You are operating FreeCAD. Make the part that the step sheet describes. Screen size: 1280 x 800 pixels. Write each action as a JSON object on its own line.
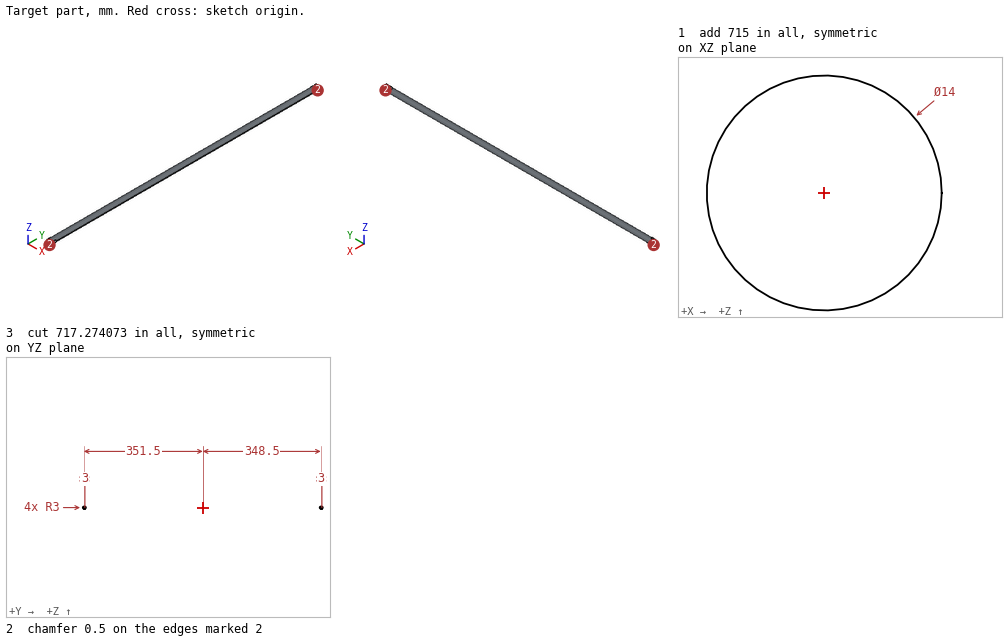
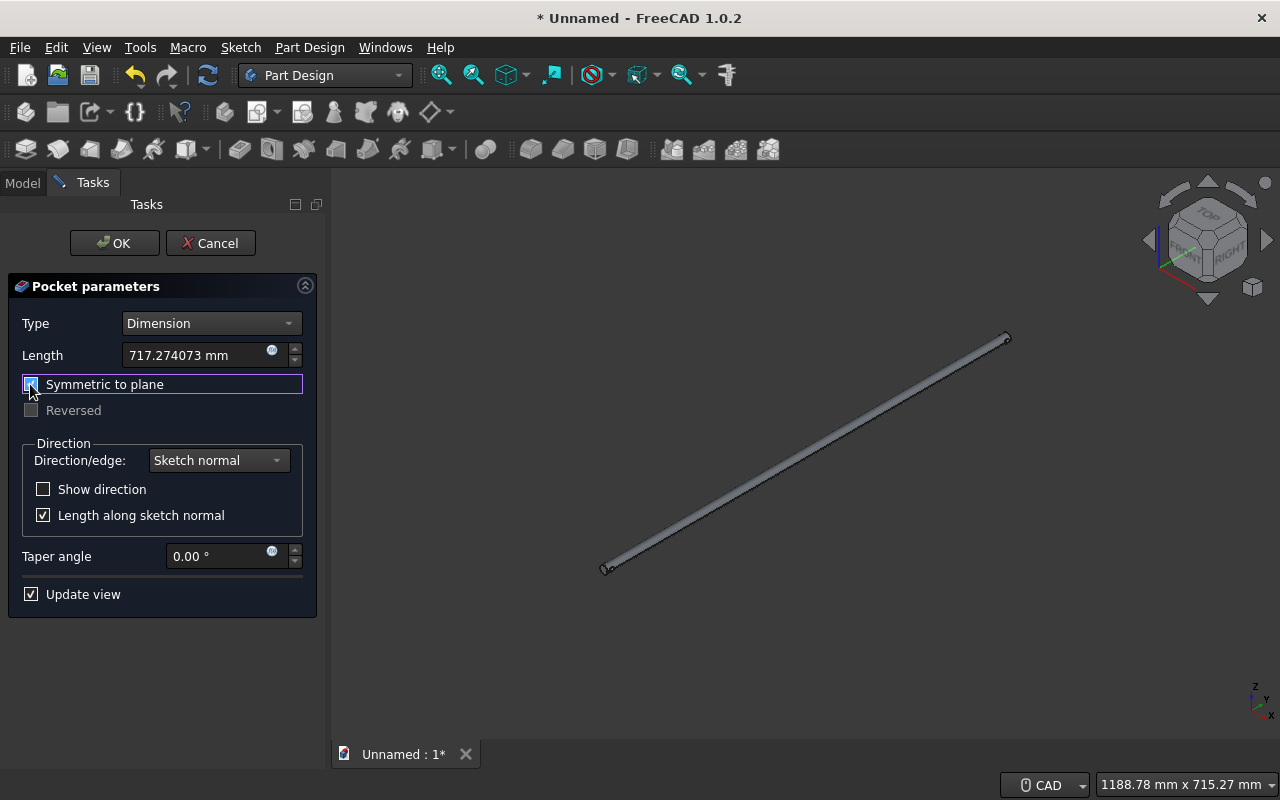
{"action": "left_click", "coordinate": [115, 243]}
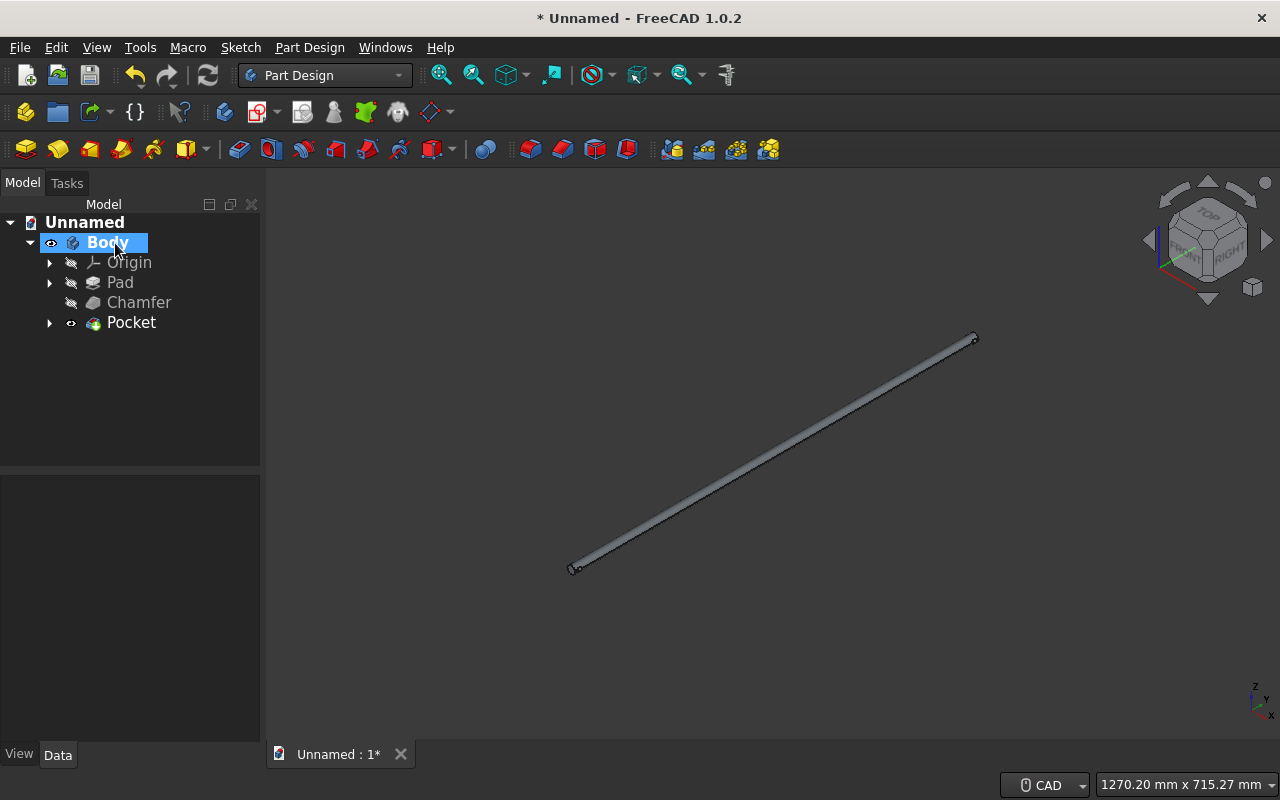
{"action": "left_click", "coordinate": [442, 76]}